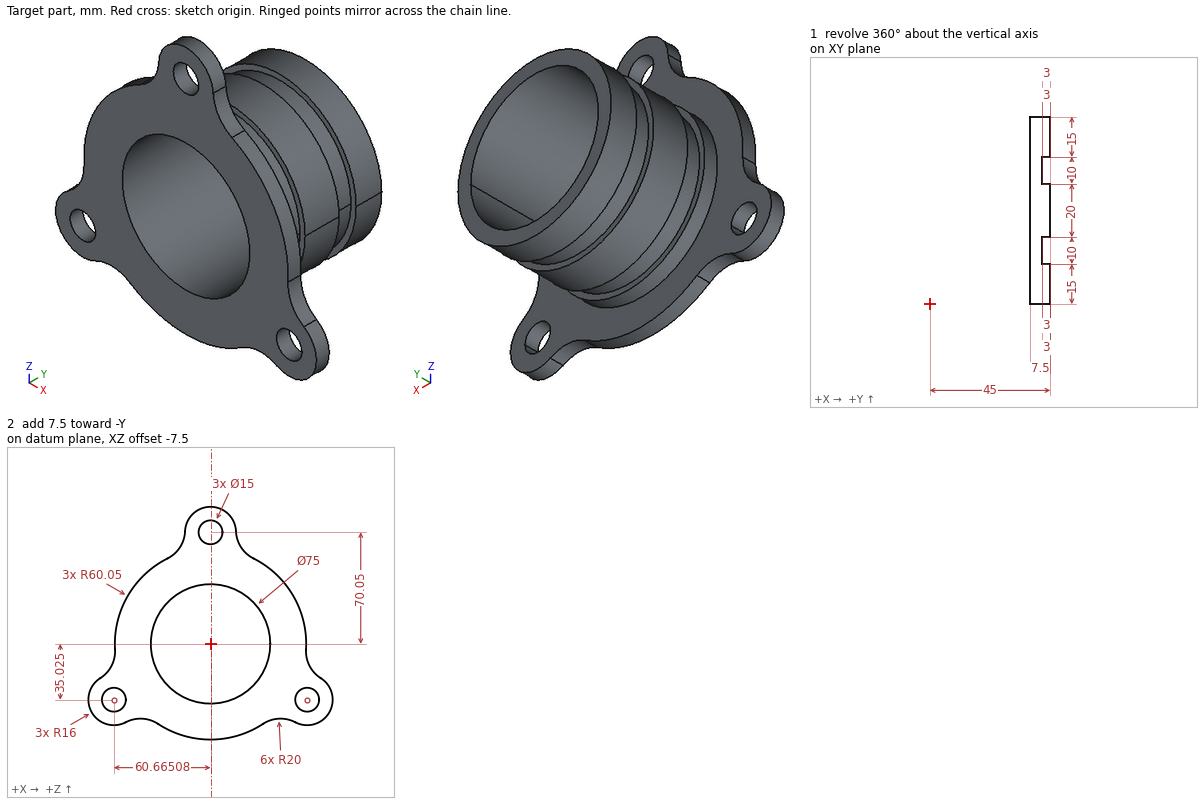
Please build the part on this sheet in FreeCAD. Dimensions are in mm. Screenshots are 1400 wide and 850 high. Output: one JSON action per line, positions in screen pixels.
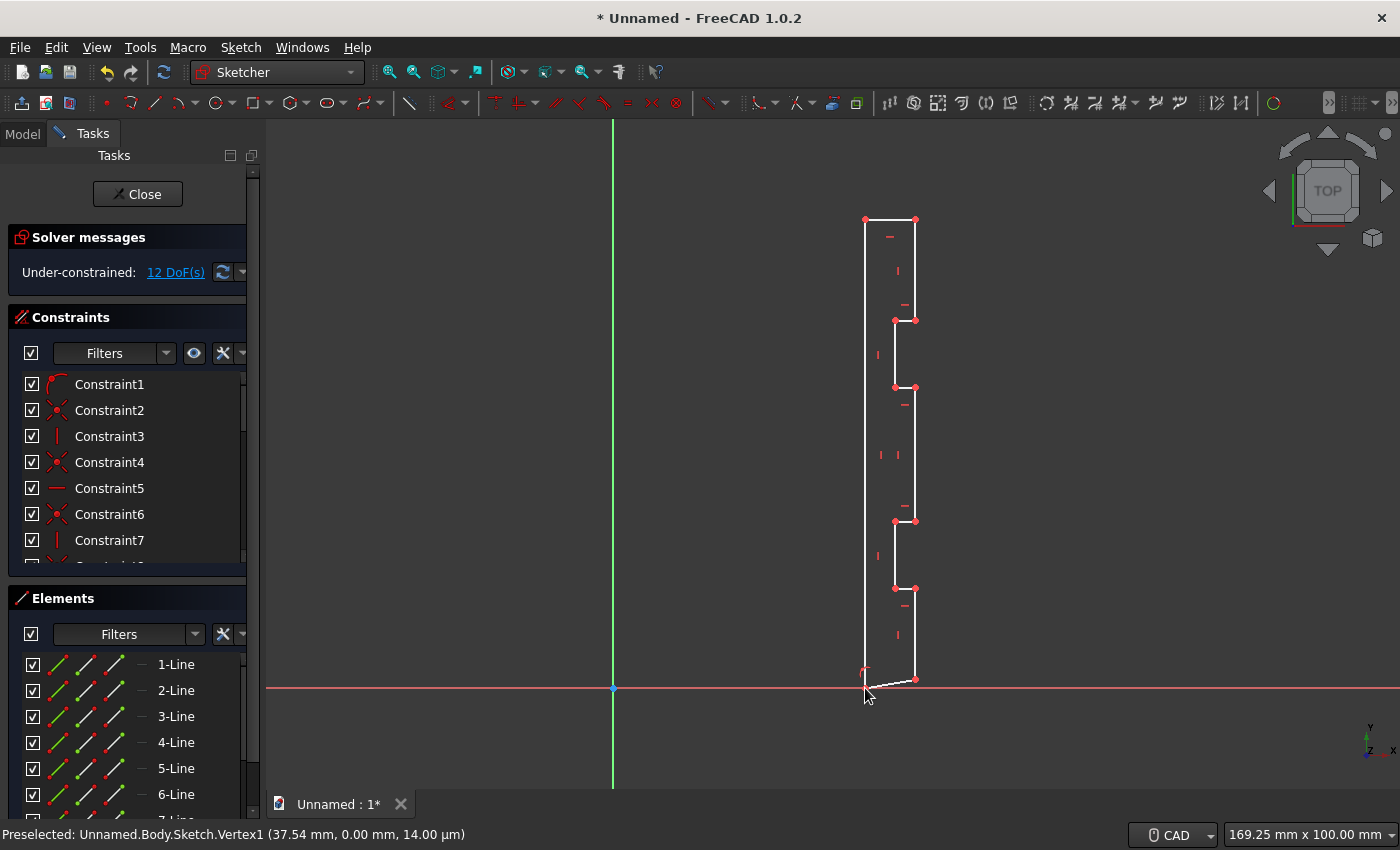
{"action": "left_click", "coordinate": [880, 686]}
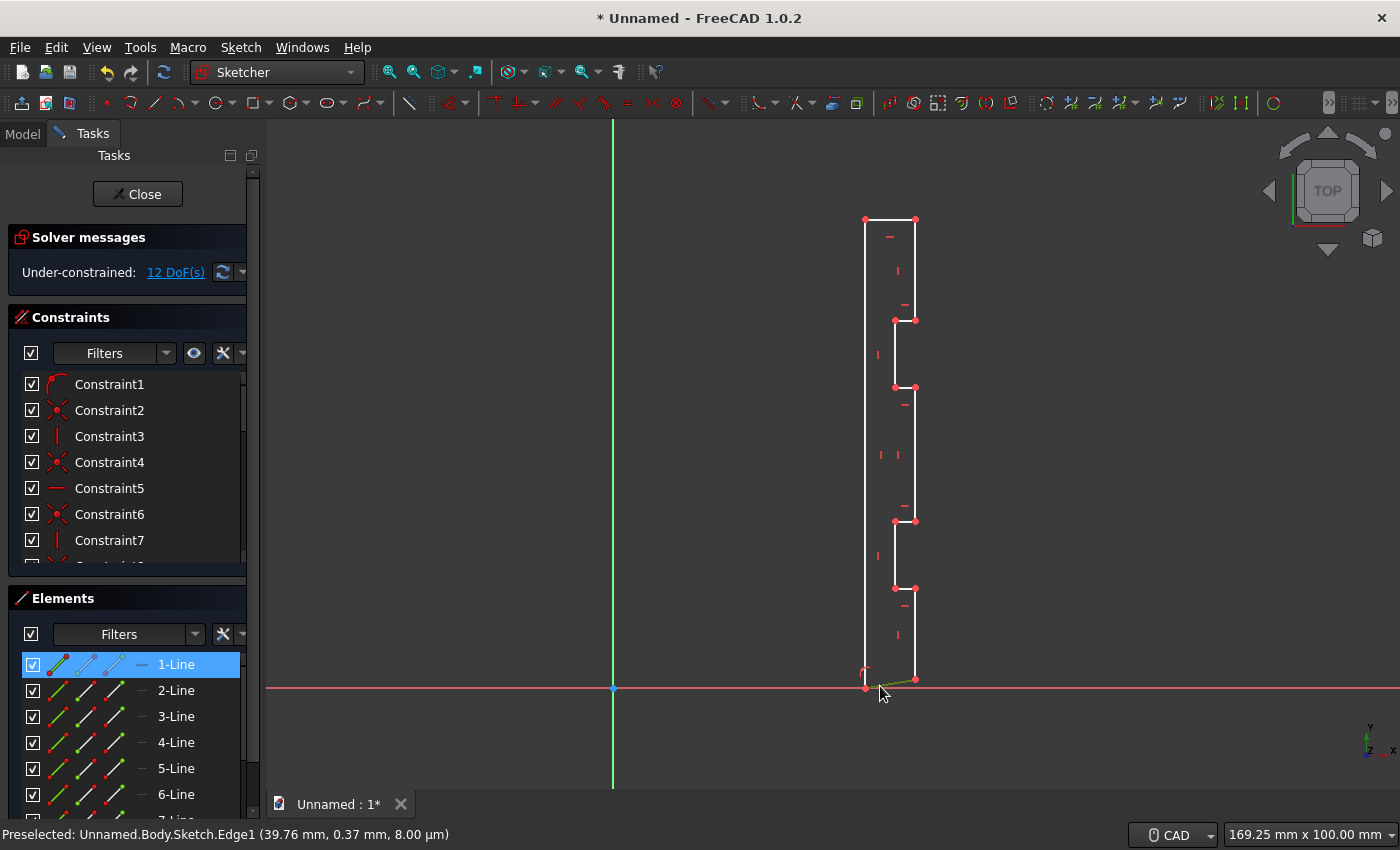
{"action": "key", "text": "h"}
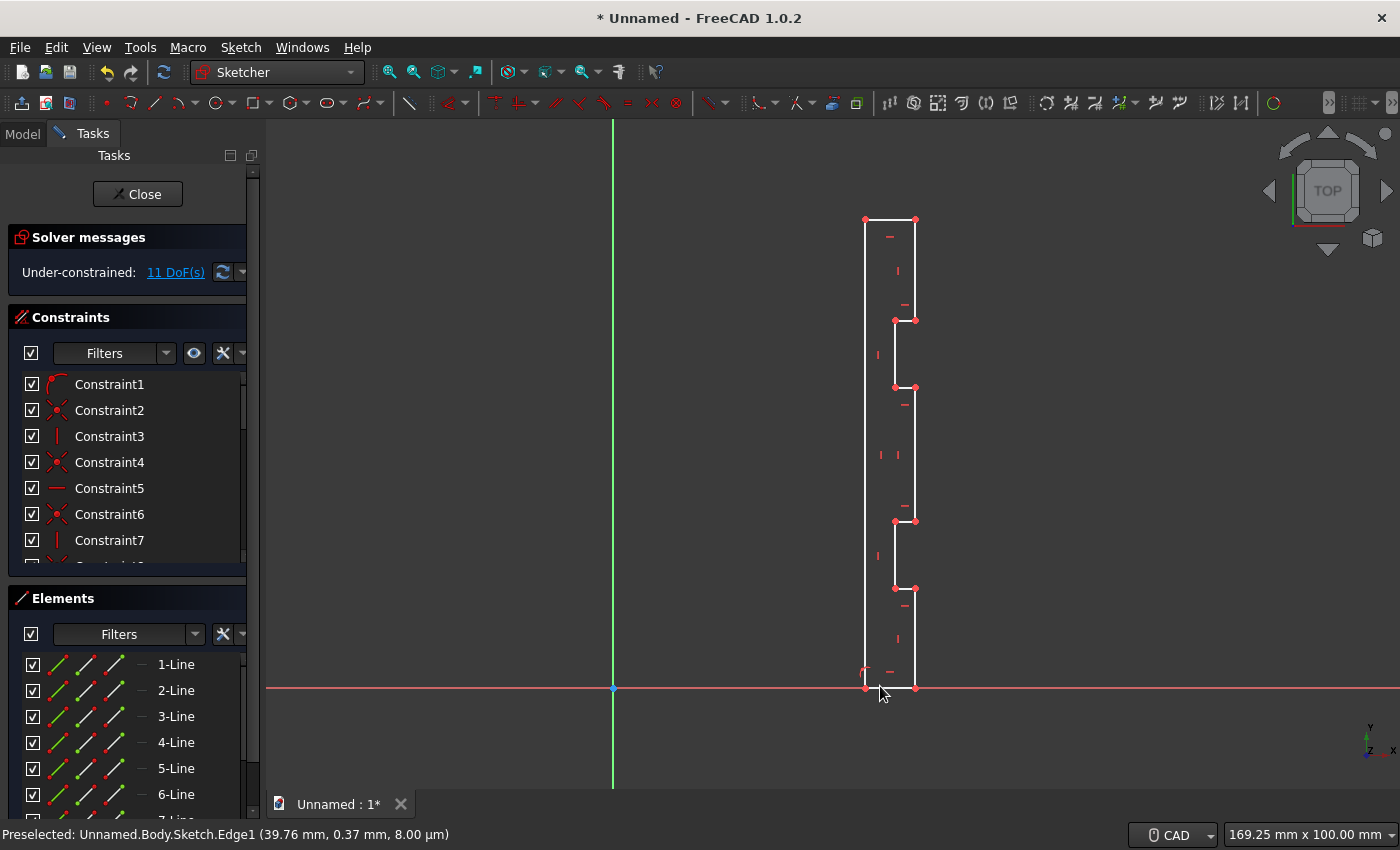
{"action": "left_click", "coordinate": [448, 104]}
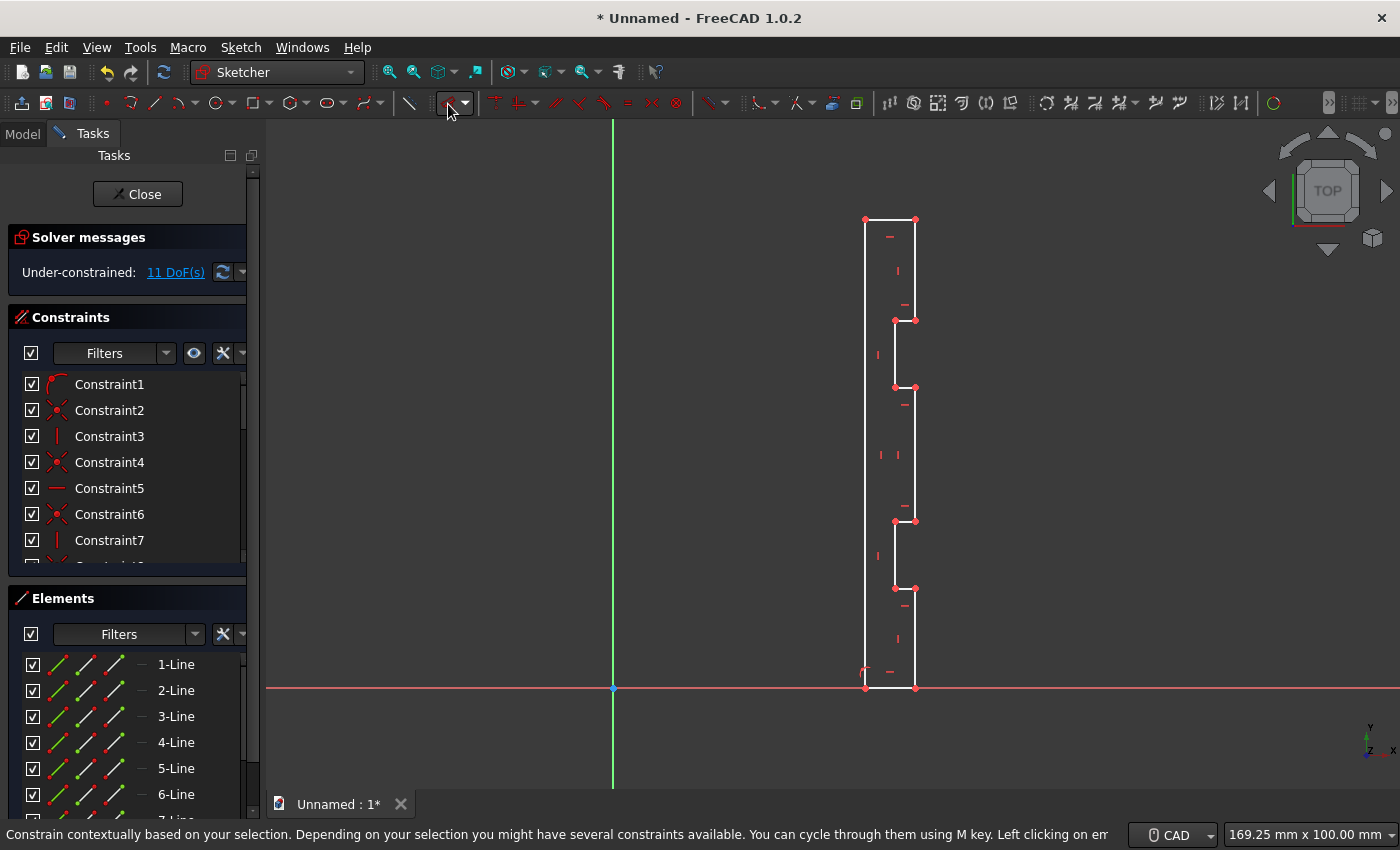
{"action": "scroll", "coordinate": [905, 589], "scroll_direction": "up", "scroll_amount": 4}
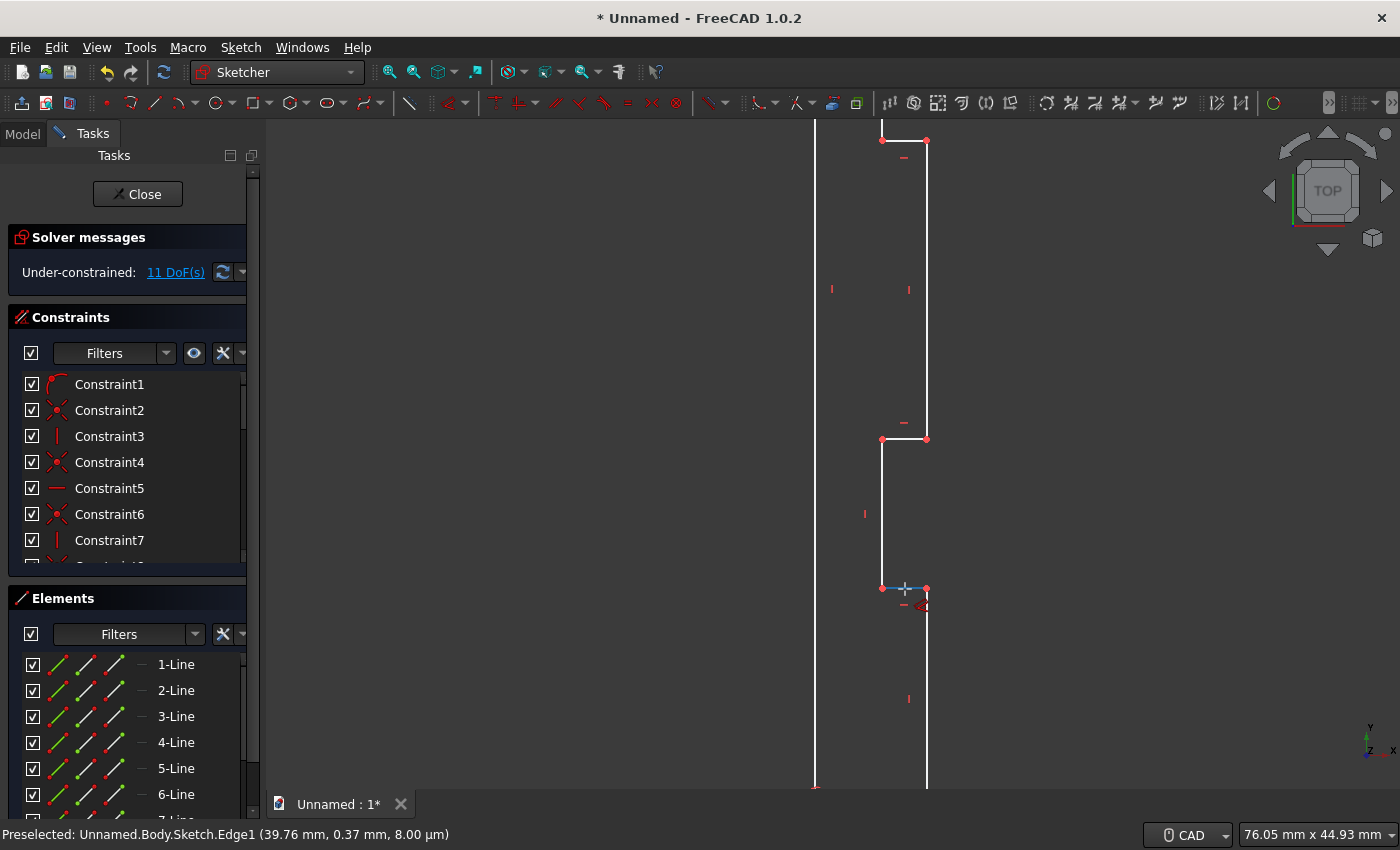
{"action": "left_click", "coordinate": [904, 588]}
{"action": "left_click", "coordinate": [904, 622]}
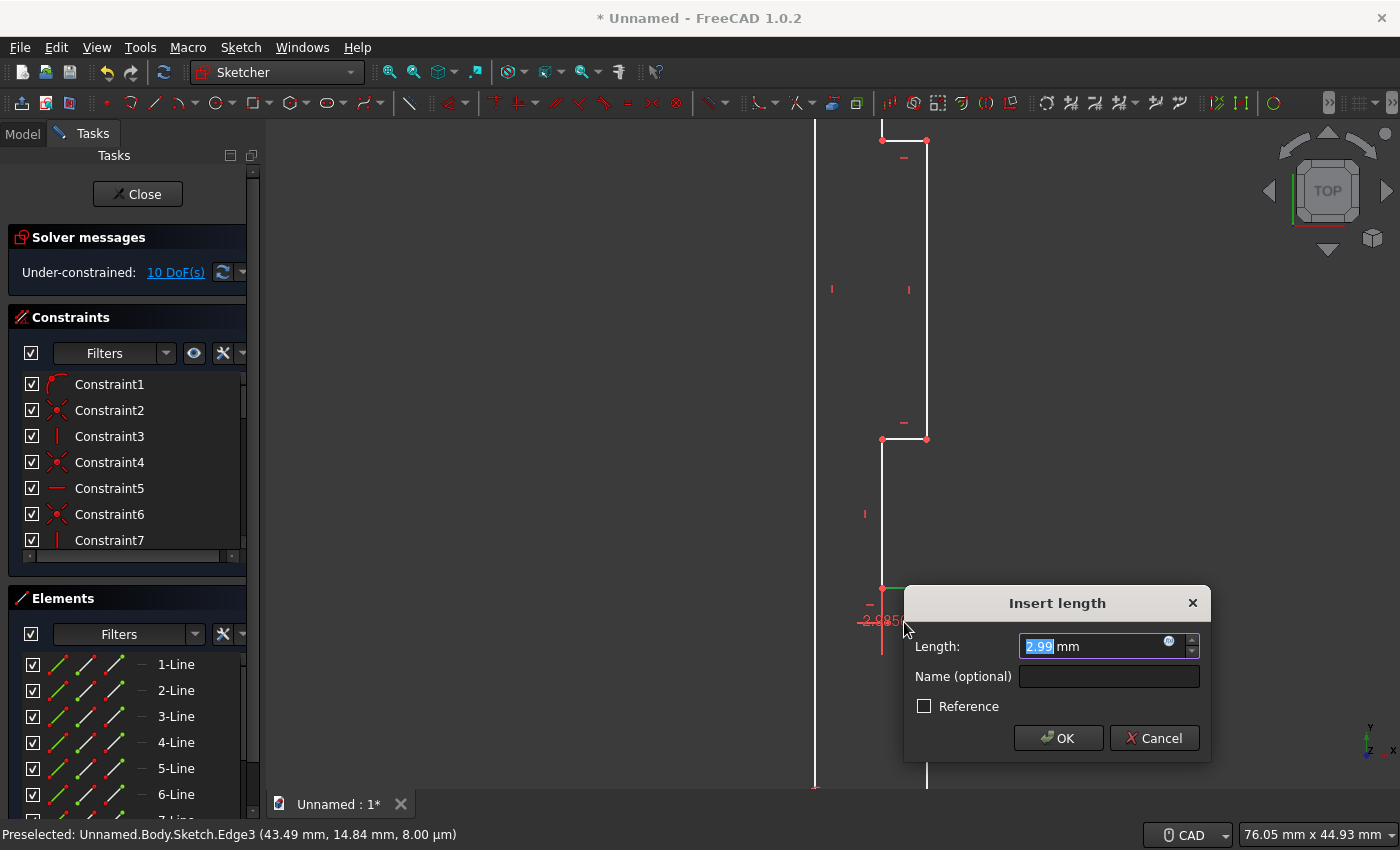
{"action": "type", "text": "3"}
{"action": "key", "text": "Return"}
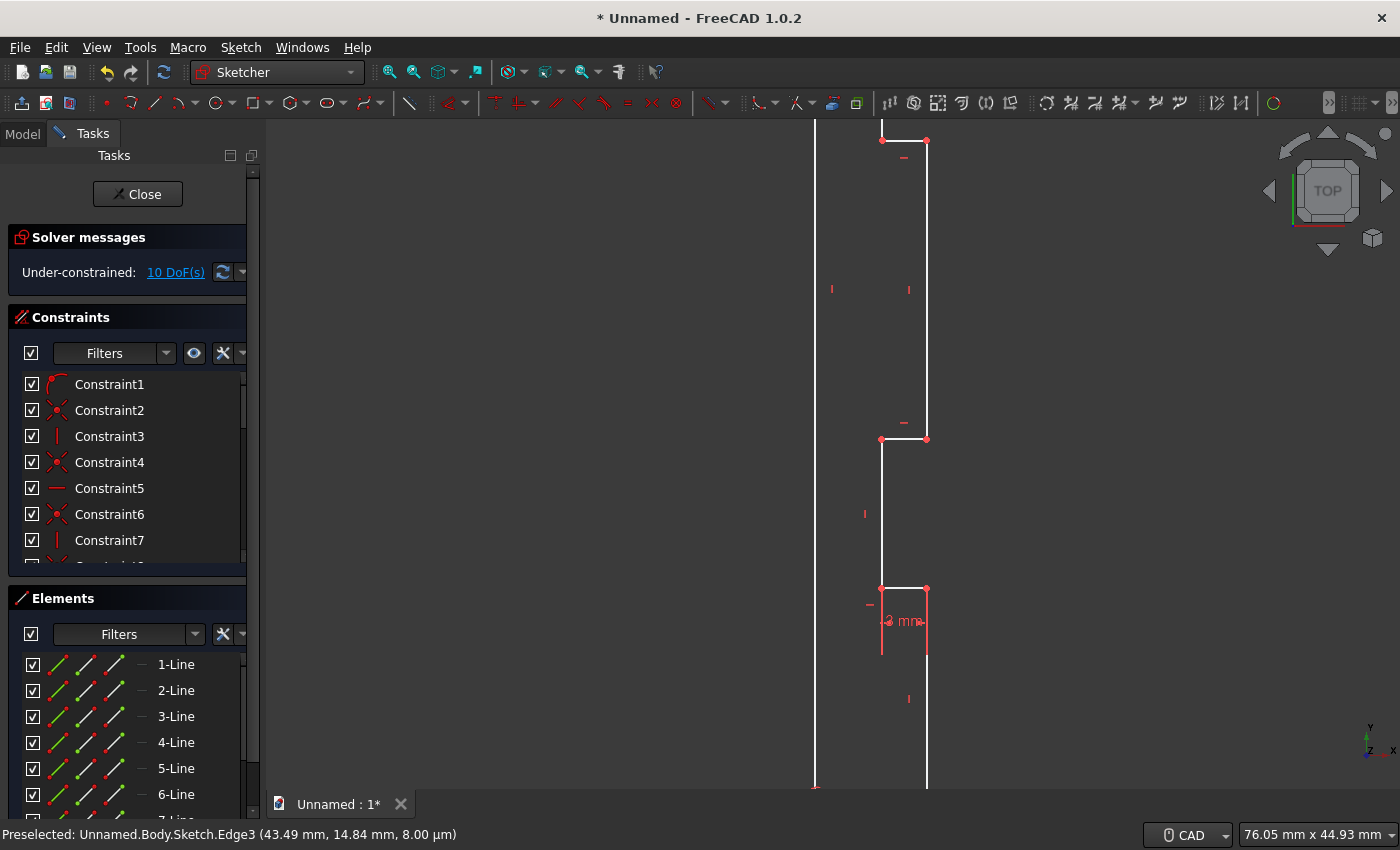
{"action": "left_click", "coordinate": [895, 439]}
{"action": "left_click", "coordinate": [904, 473]}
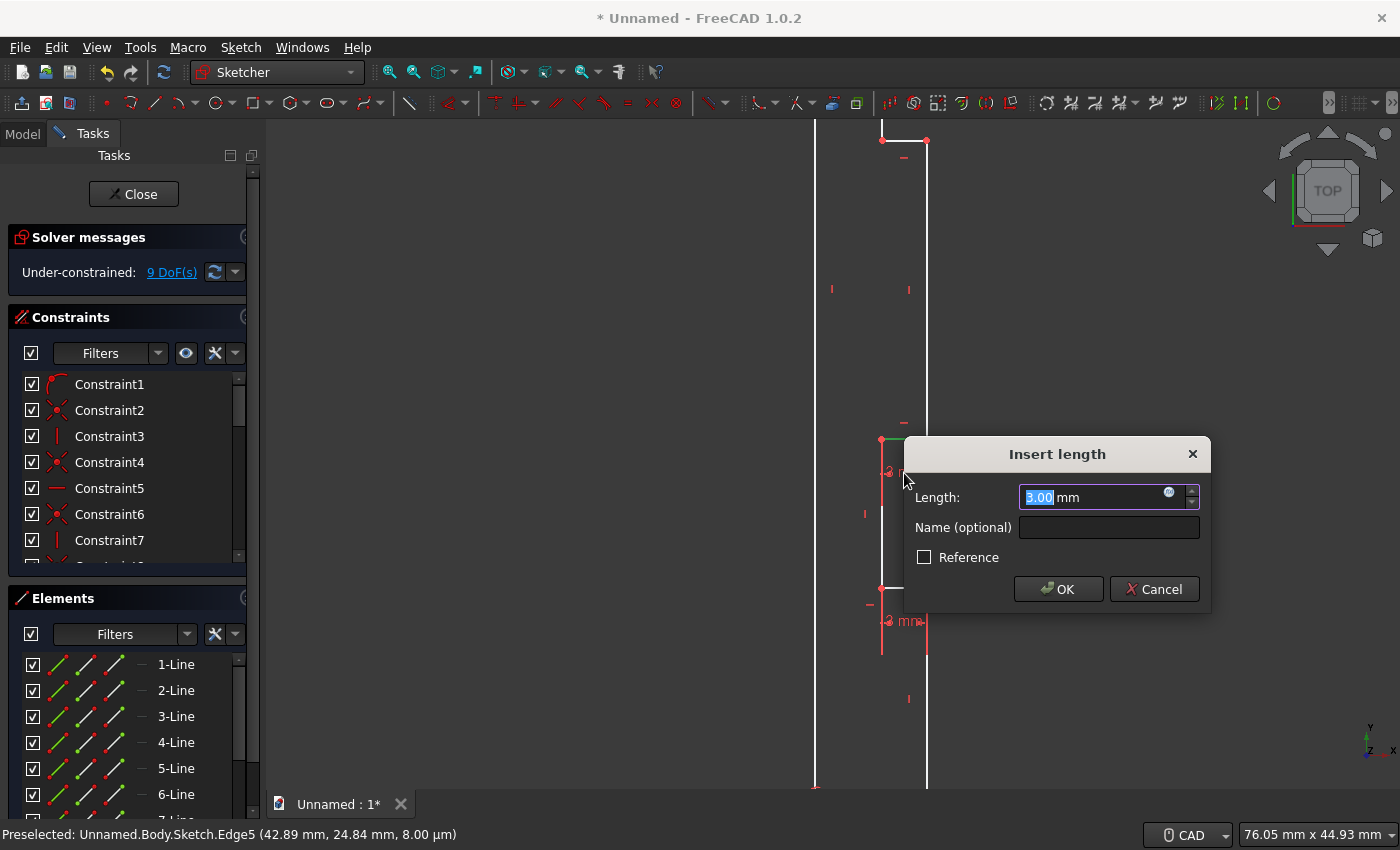
{"action": "type", "text": "3"}
{"action": "key", "text": "Return"}